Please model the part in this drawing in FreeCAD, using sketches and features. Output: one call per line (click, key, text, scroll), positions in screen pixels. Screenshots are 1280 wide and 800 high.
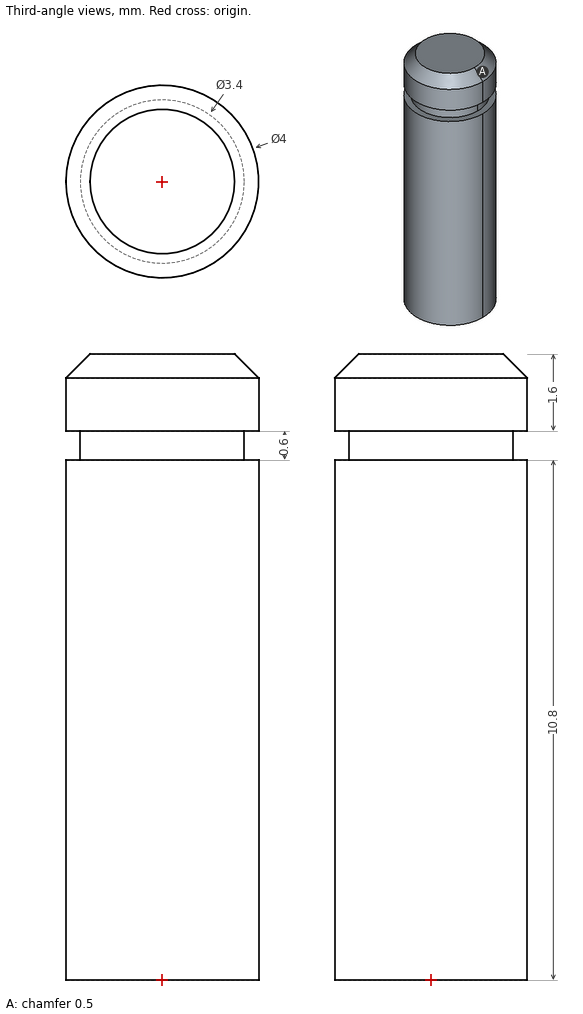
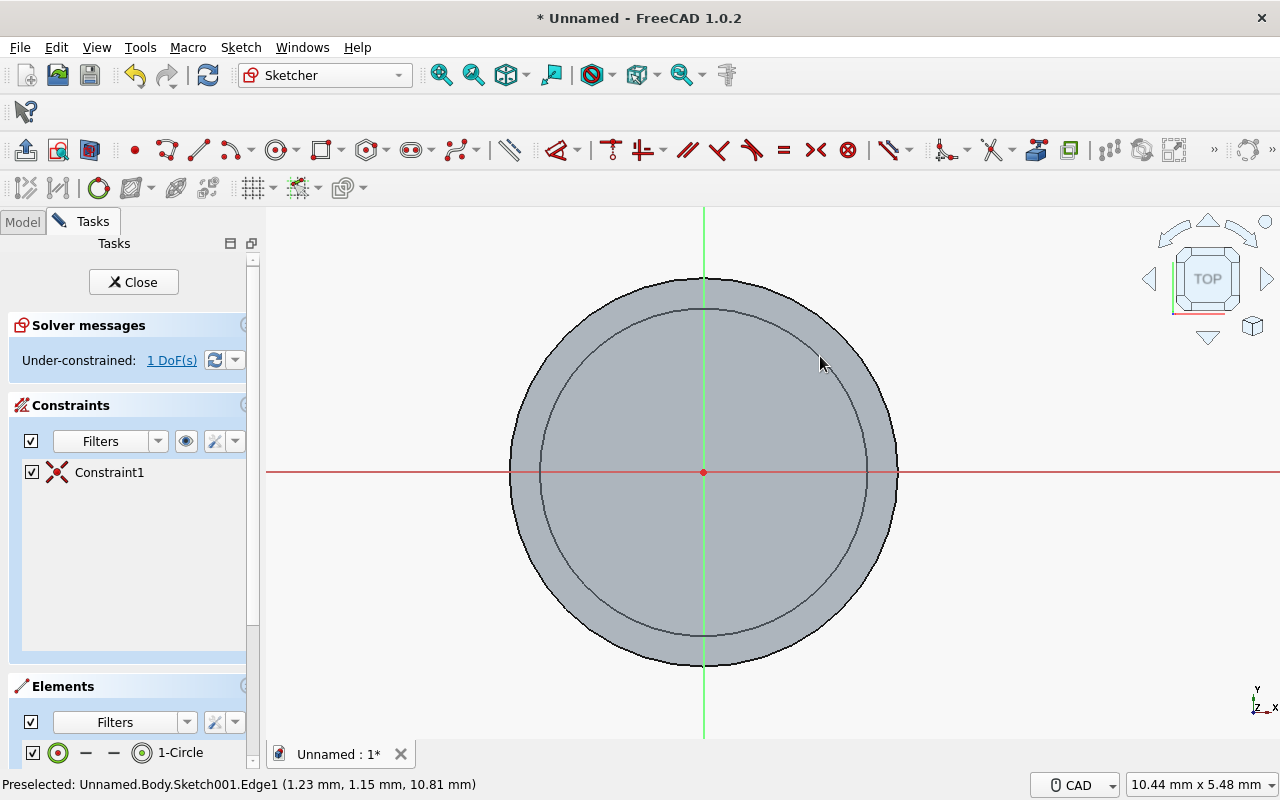
key(d)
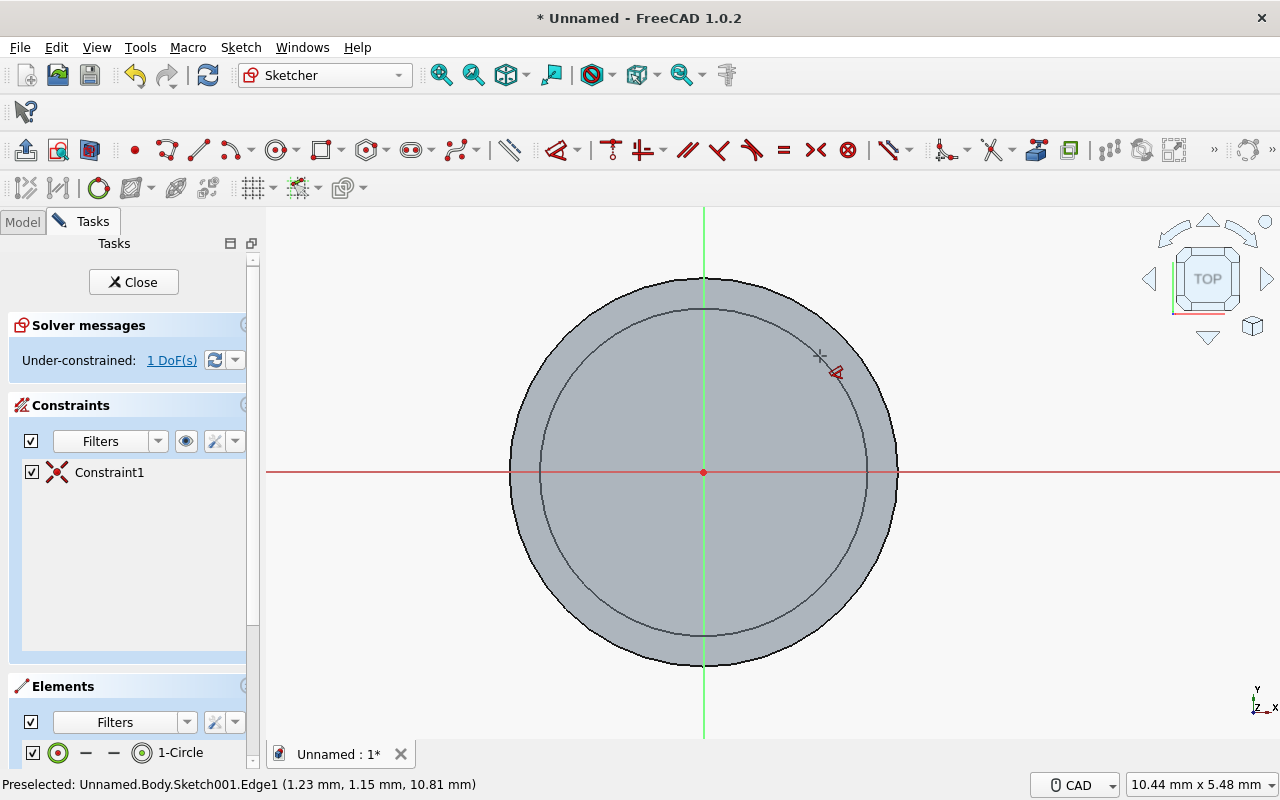
click(819, 356)
click(842, 333)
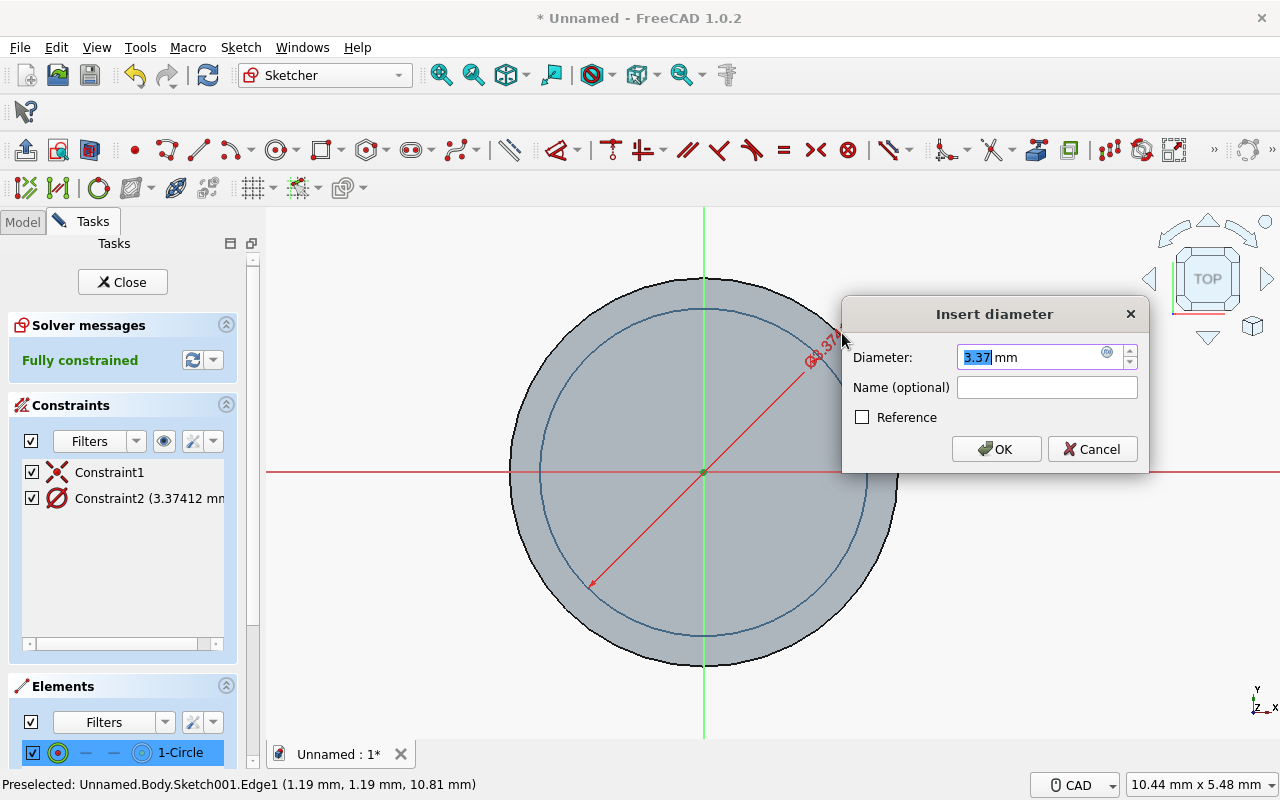
text(3.4)
key(Return)
key(Escape)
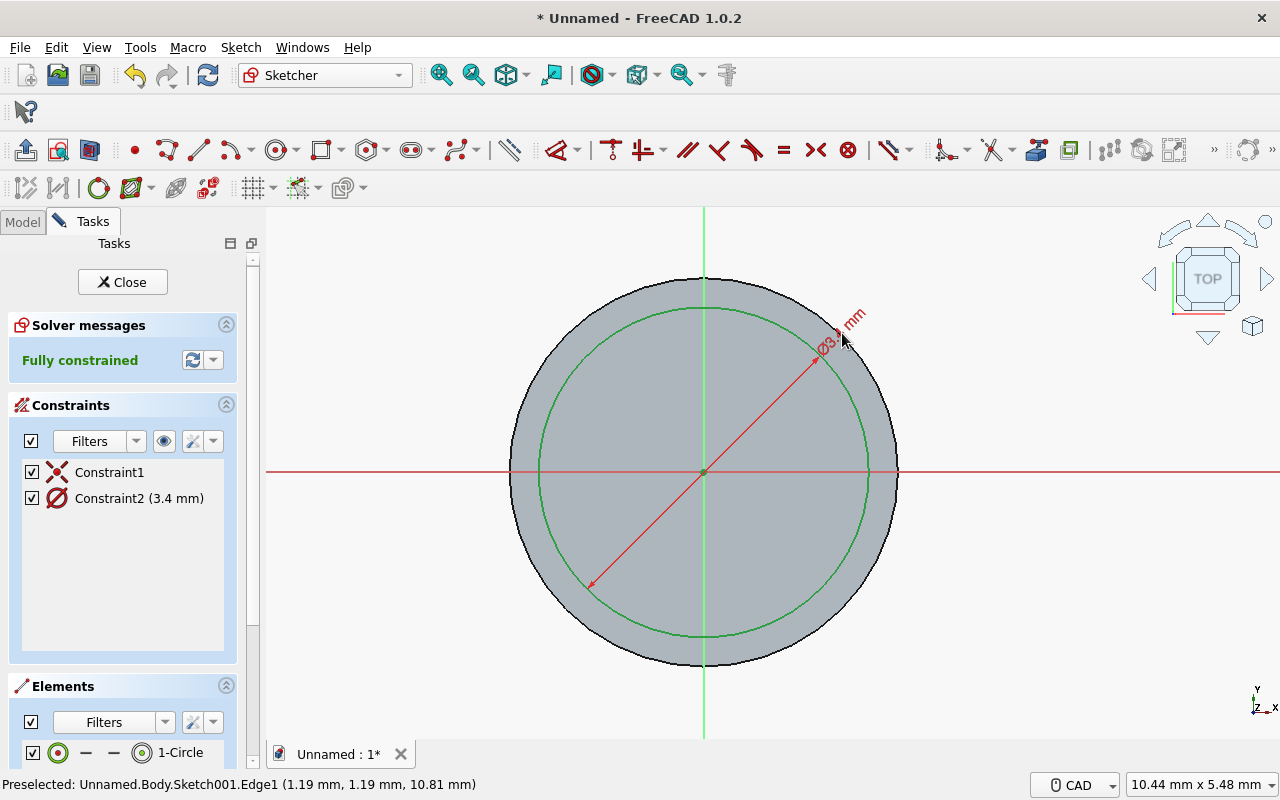
click(123, 282)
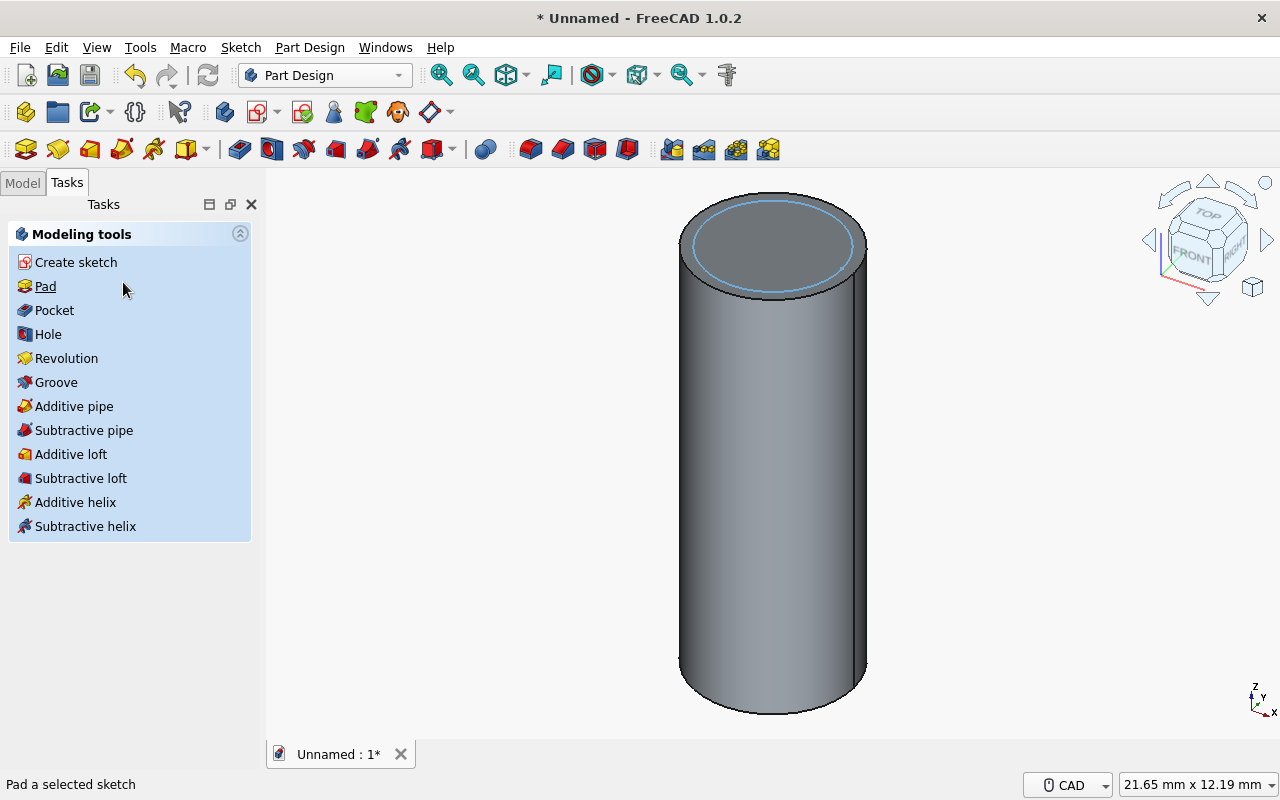
click(26, 150)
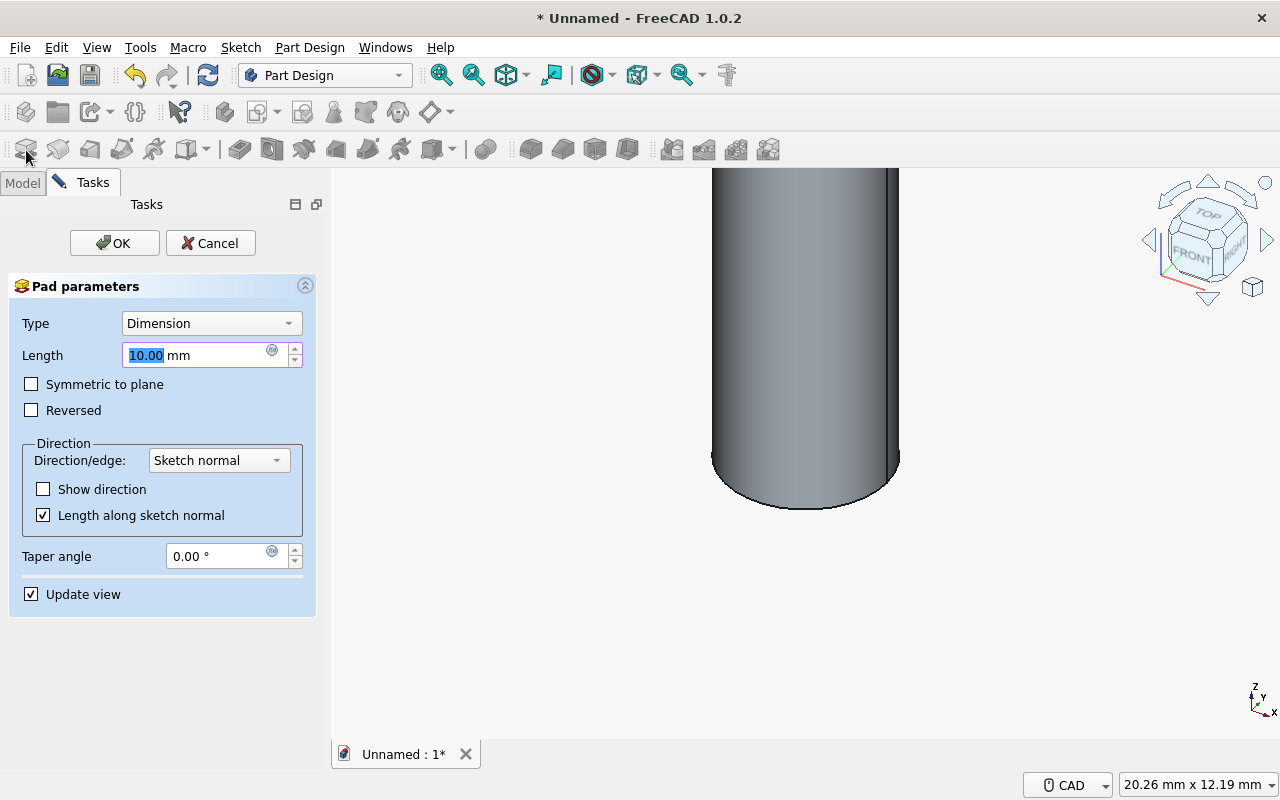
text(0.6)
key(Tab)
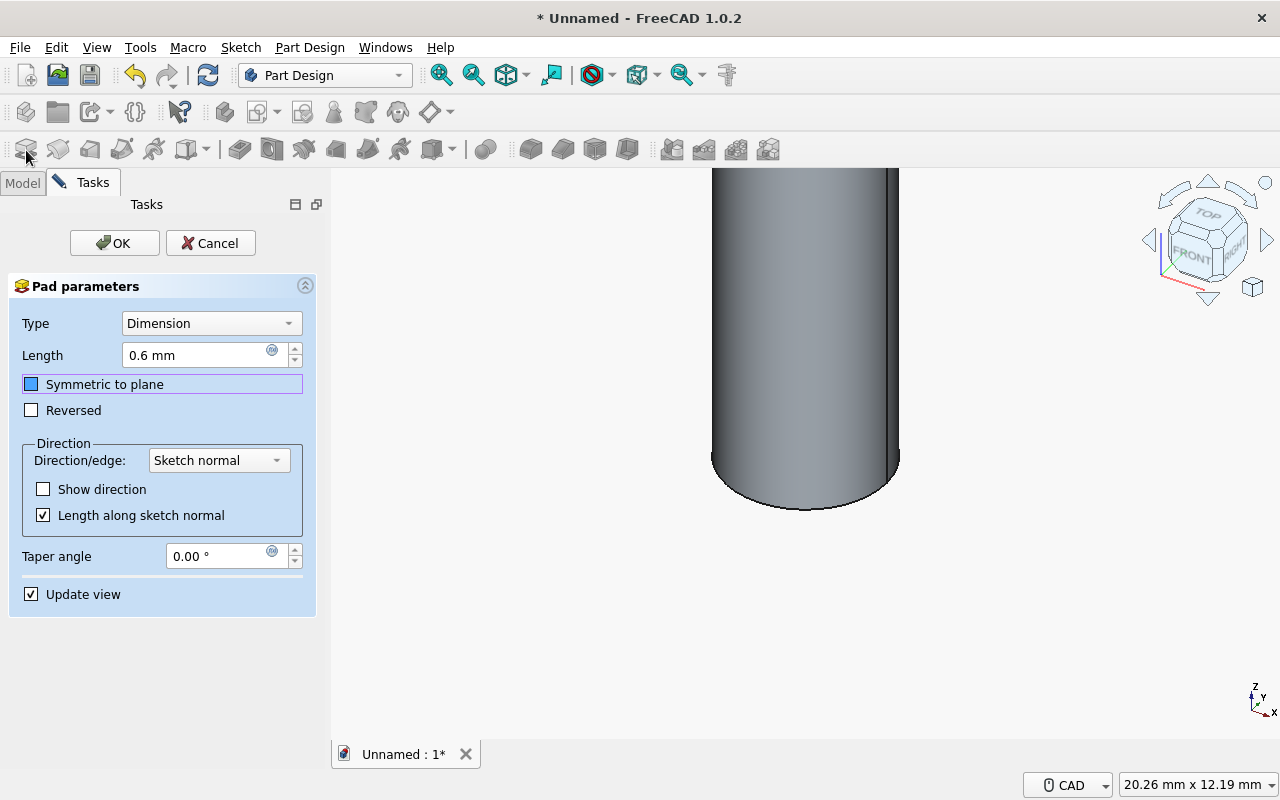
click(115, 243)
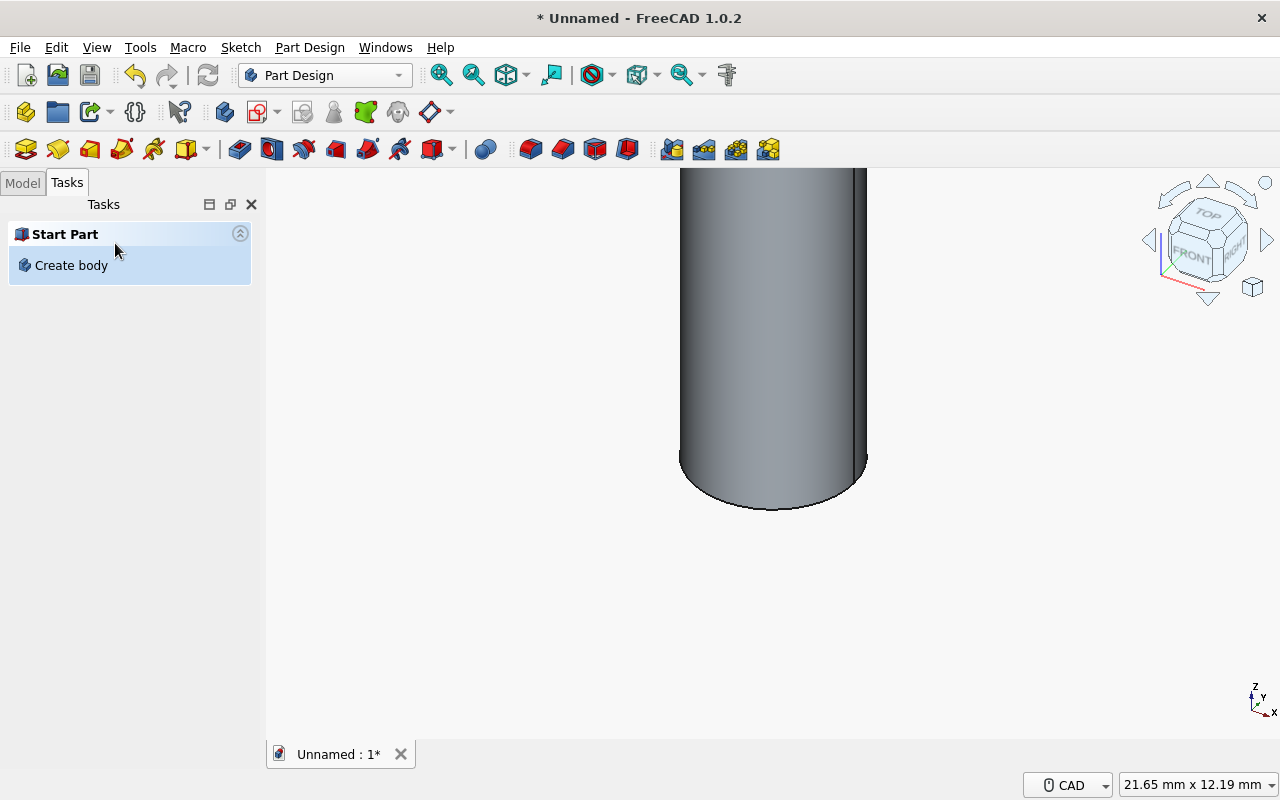
key(v)
key(f)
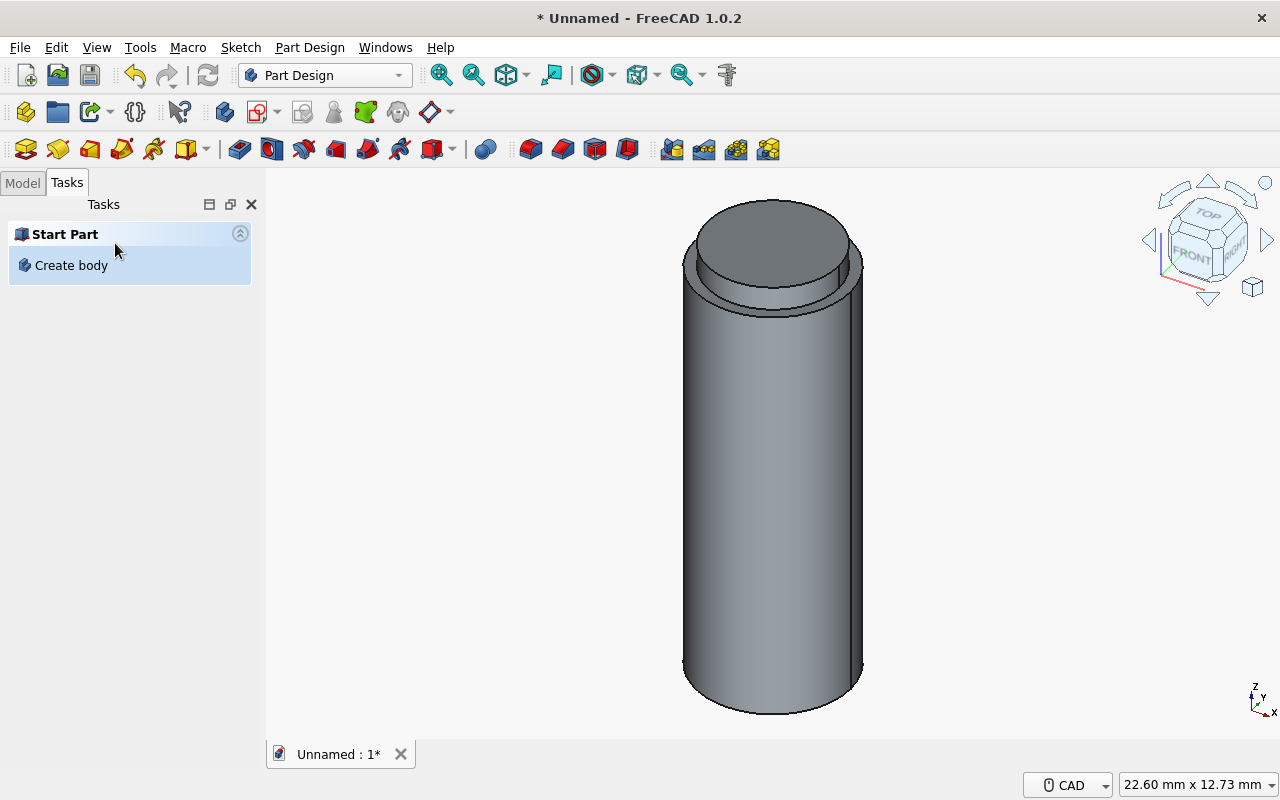
click(773, 243)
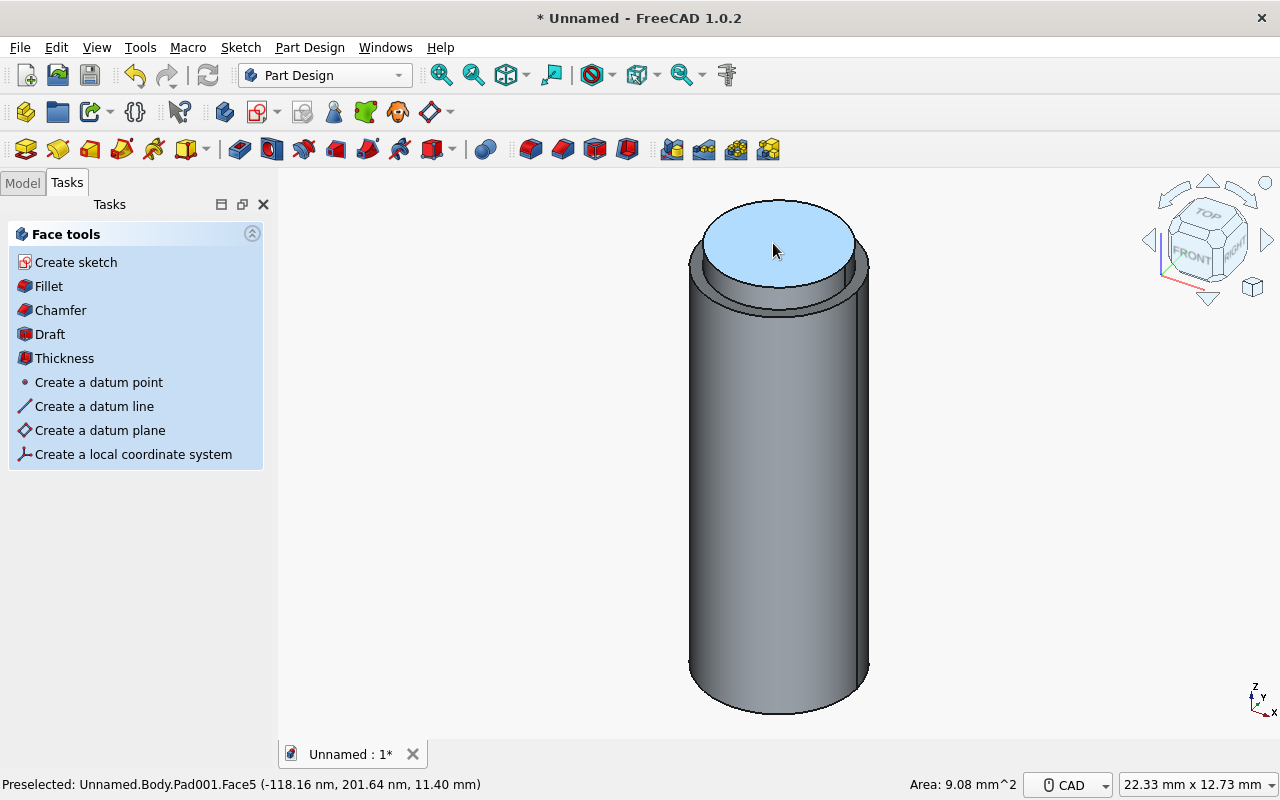
click(258, 112)